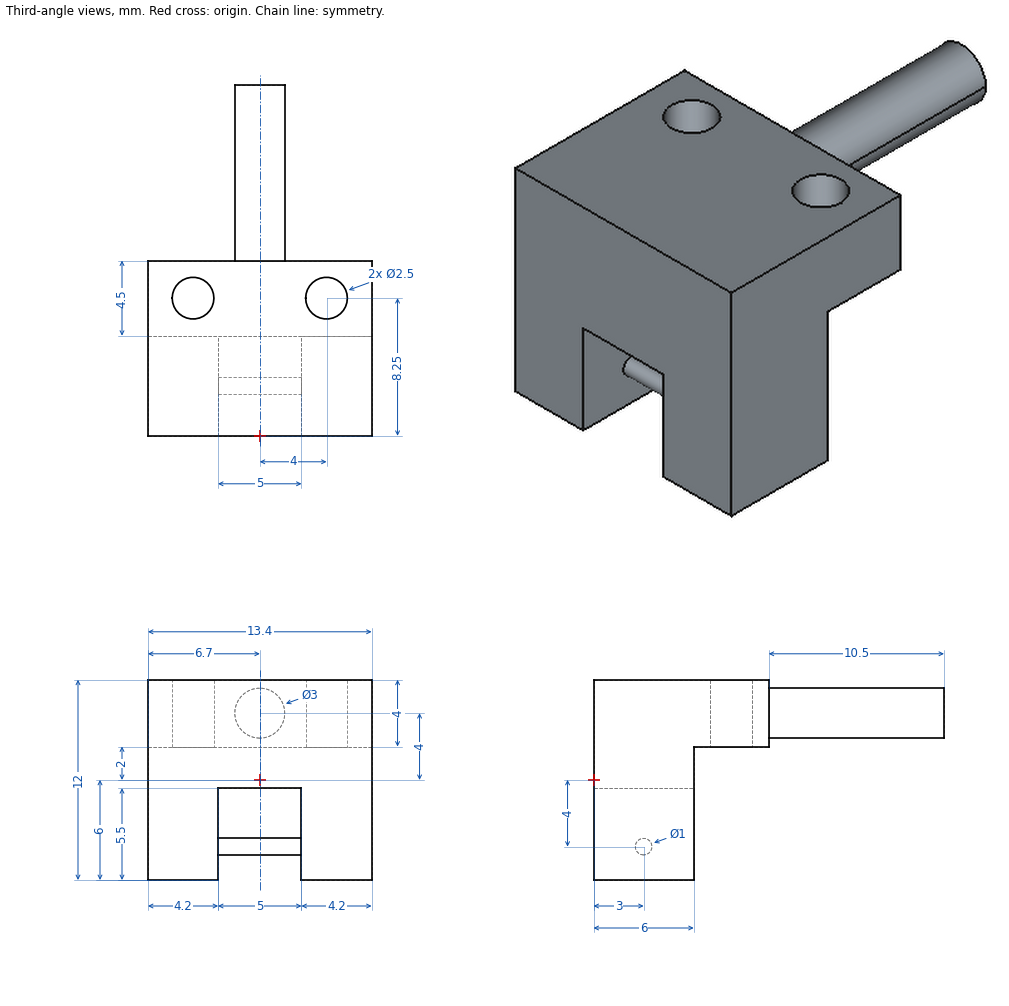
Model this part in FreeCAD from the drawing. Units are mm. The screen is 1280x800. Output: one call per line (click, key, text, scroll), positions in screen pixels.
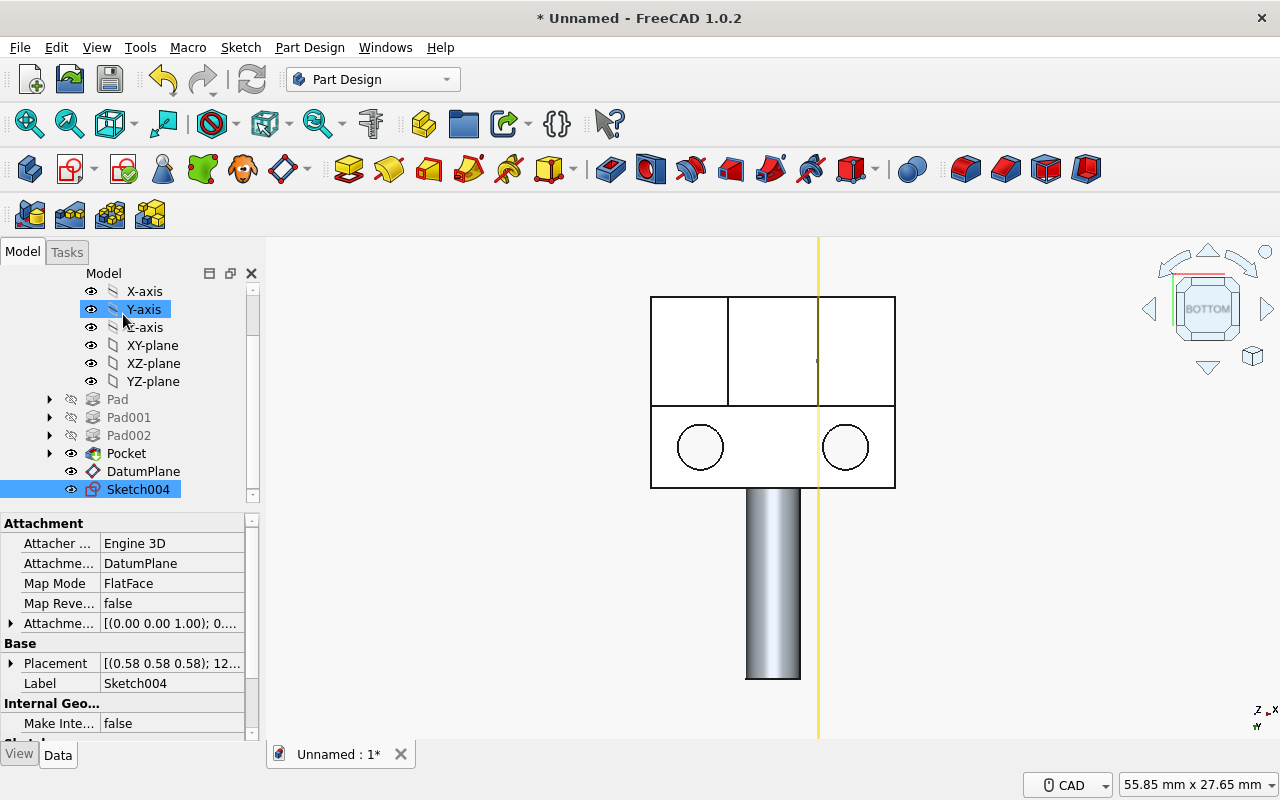
click(350, 170)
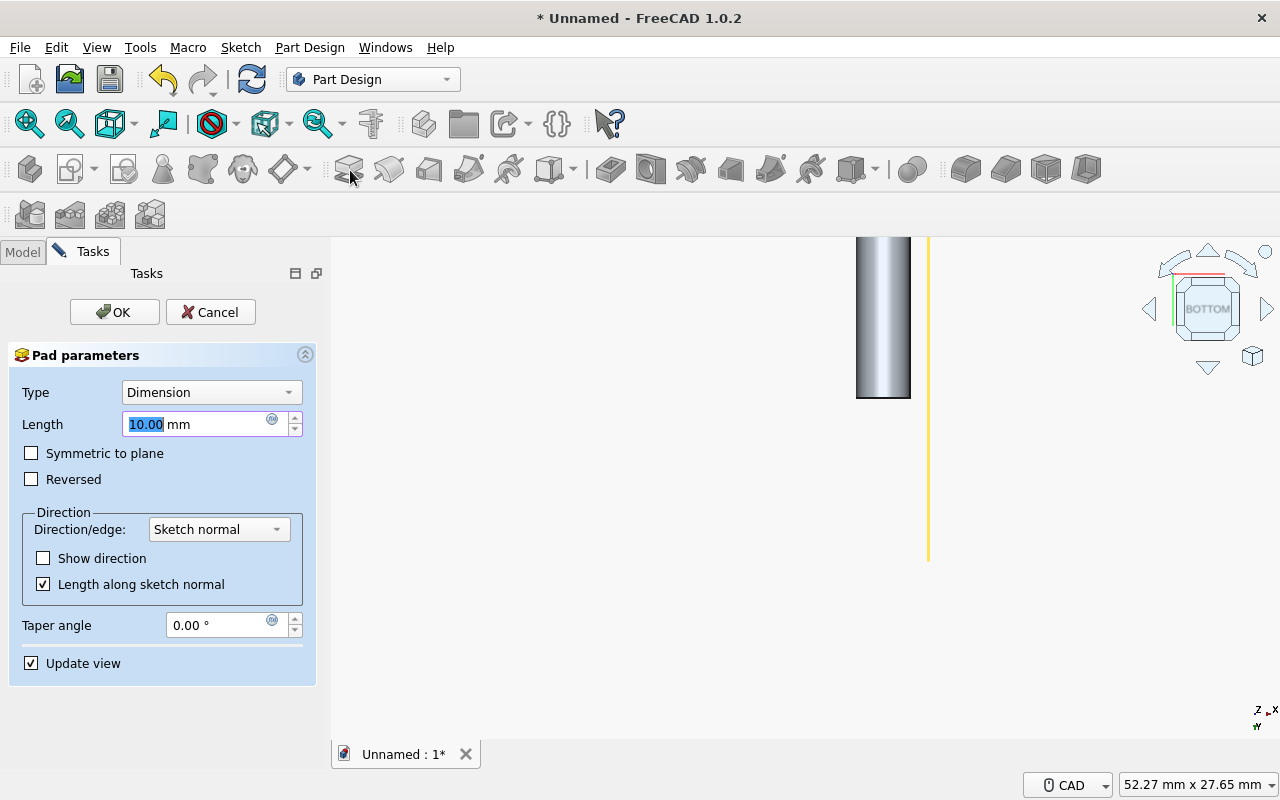
text(5)
key(Tab)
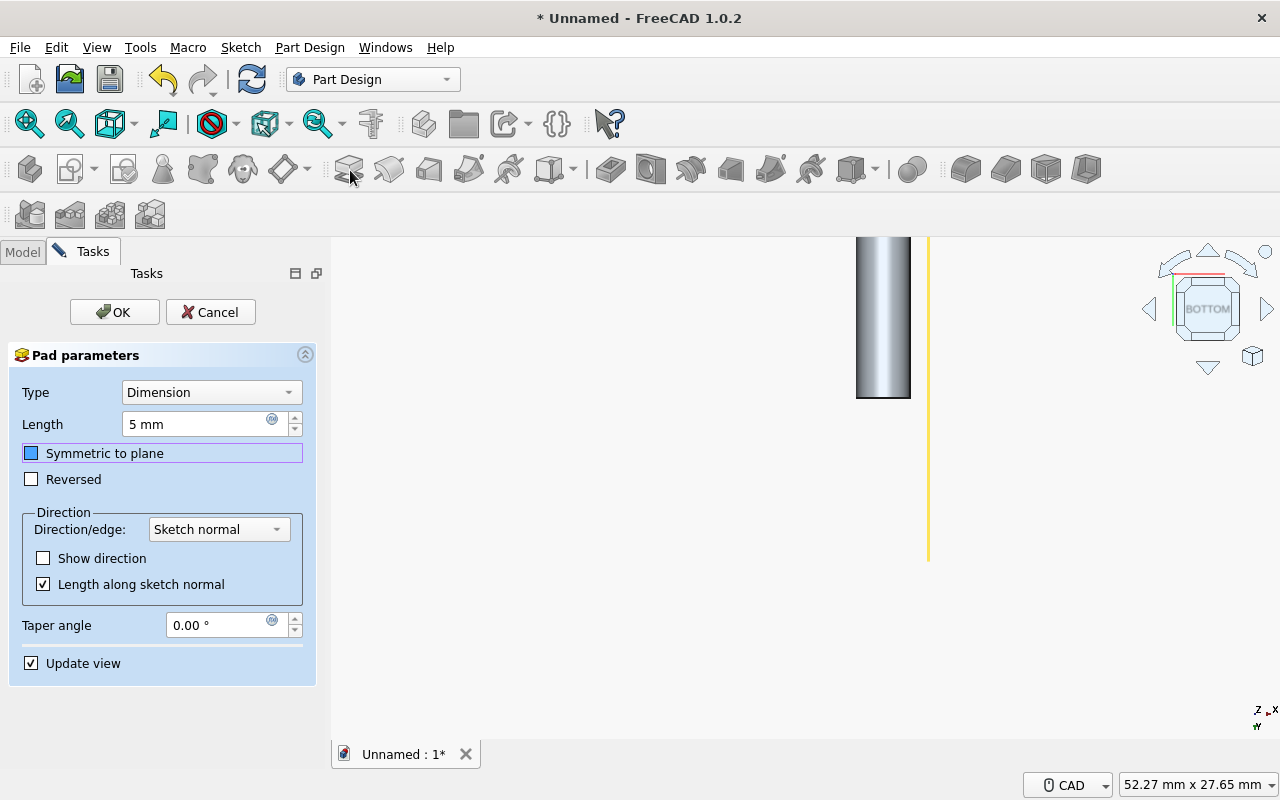
click(30, 479)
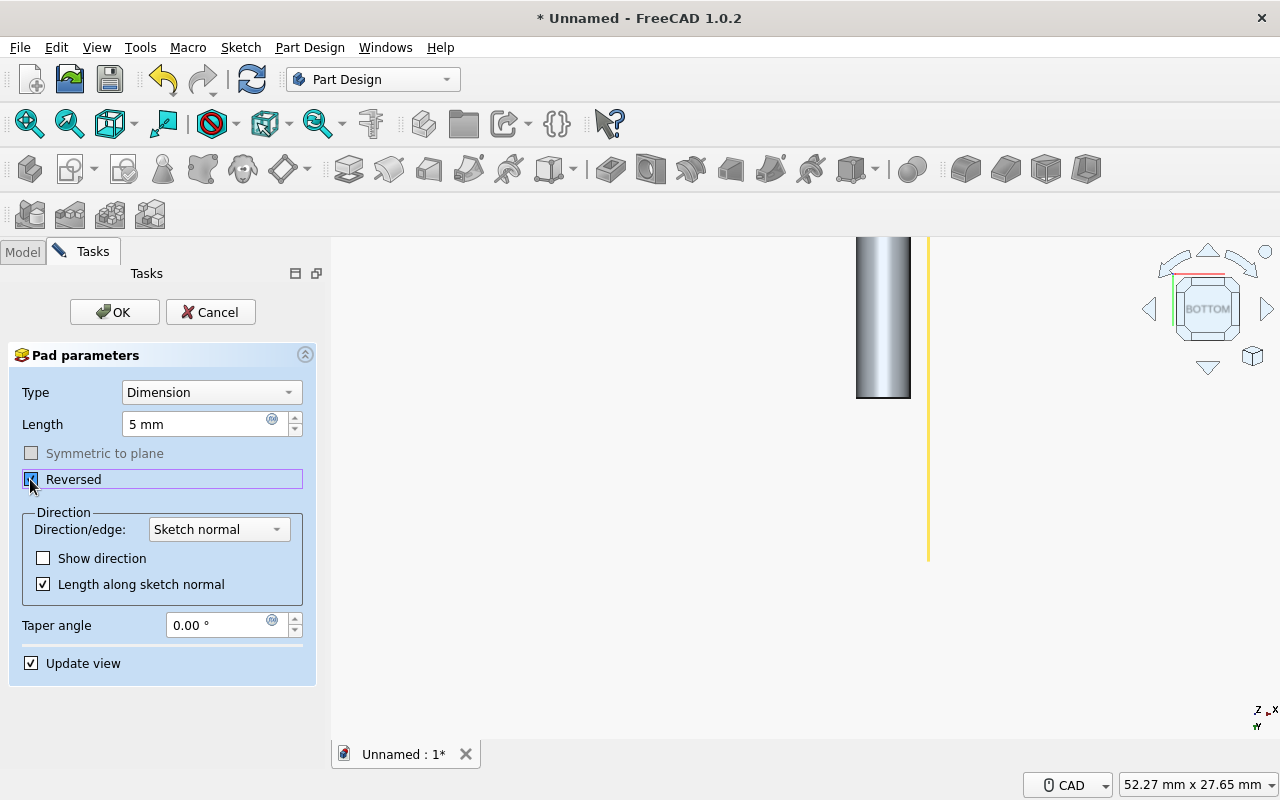
click(115, 312)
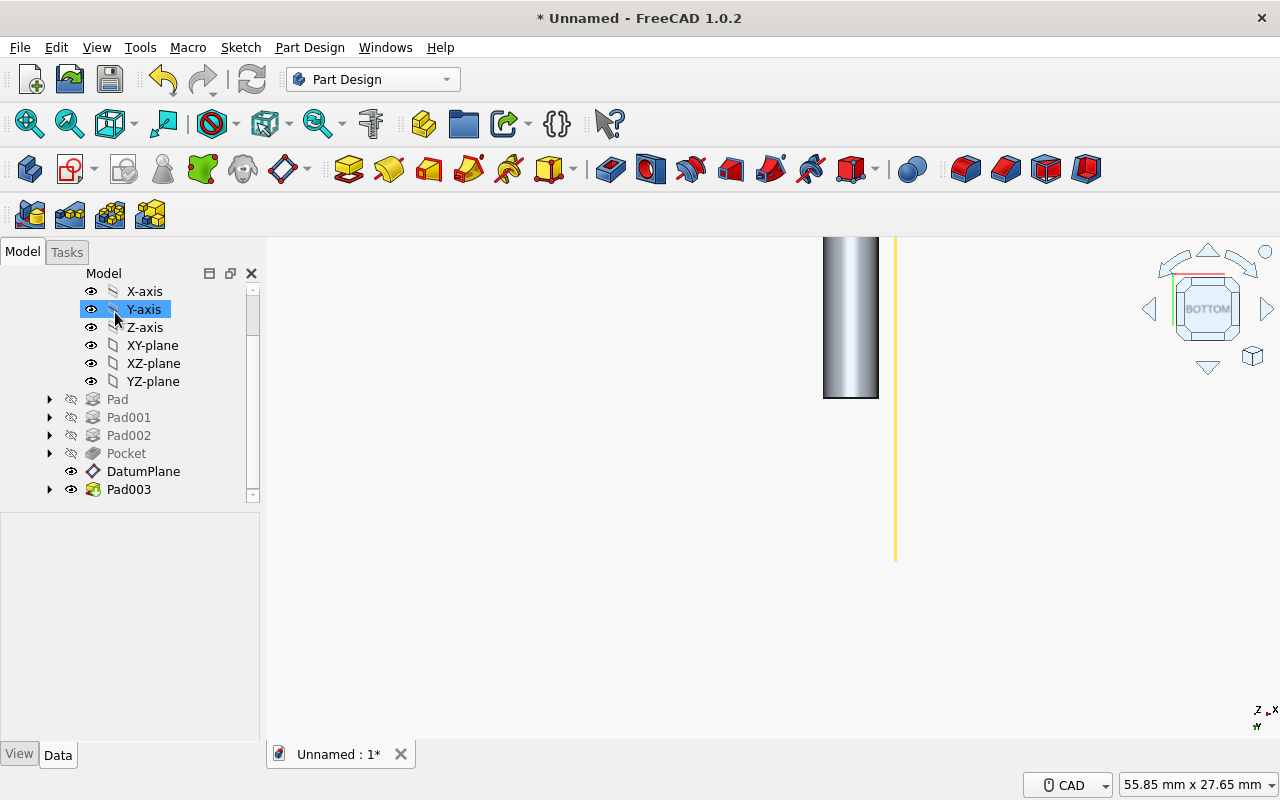
click(116, 471)
key(space)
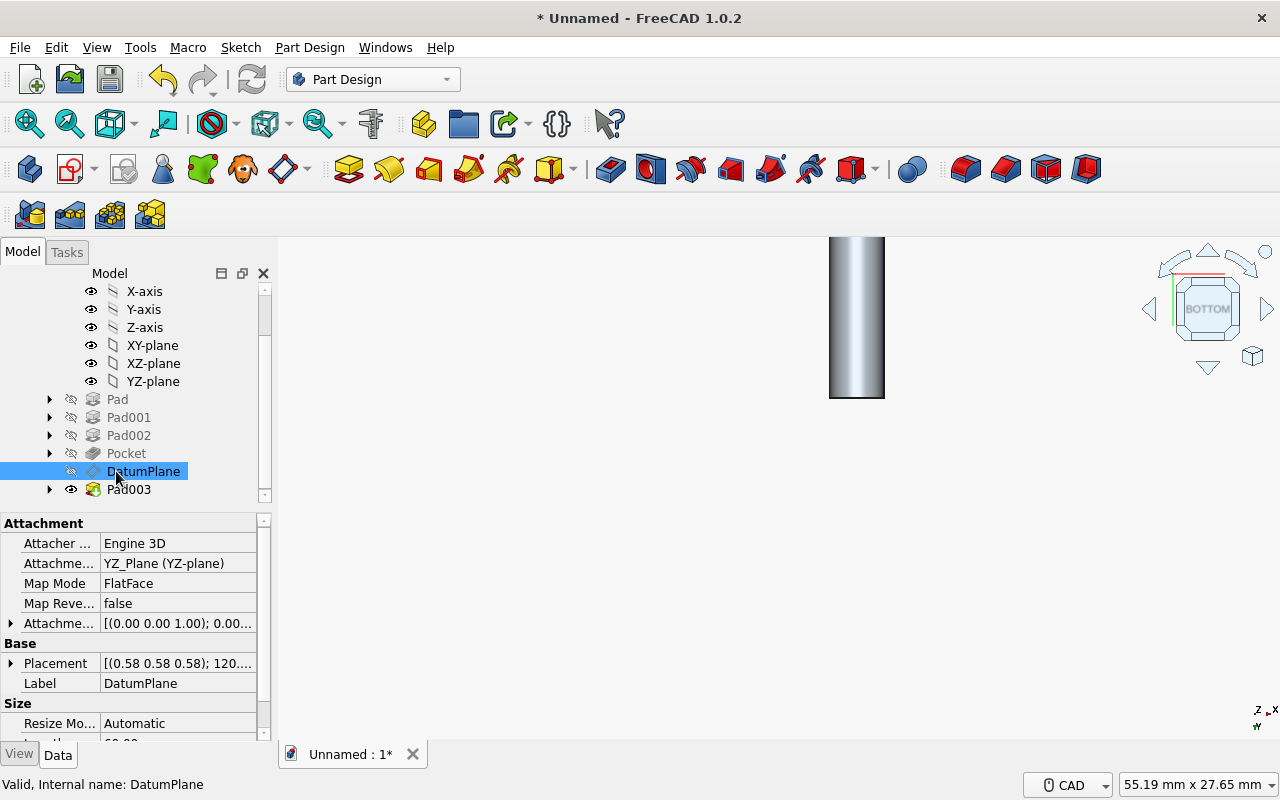
key(0)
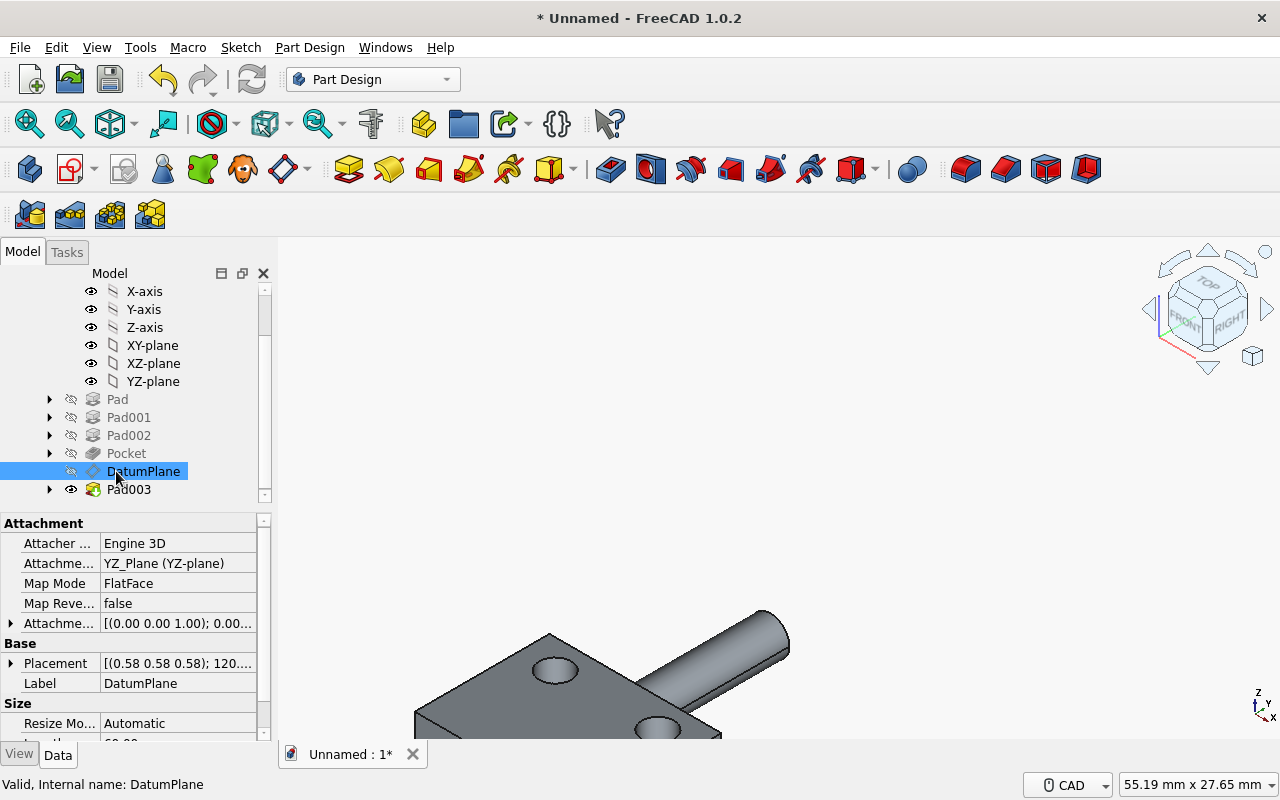
click(30, 124)